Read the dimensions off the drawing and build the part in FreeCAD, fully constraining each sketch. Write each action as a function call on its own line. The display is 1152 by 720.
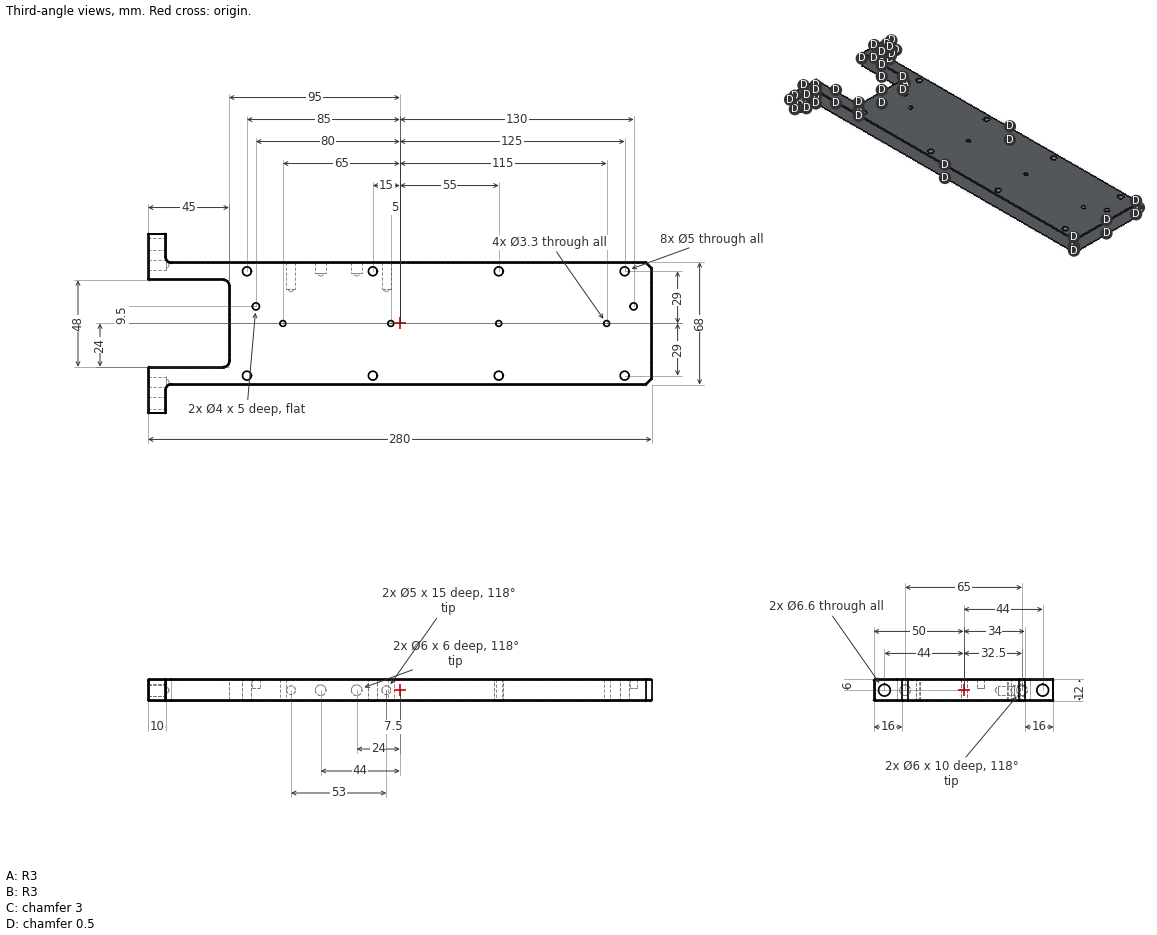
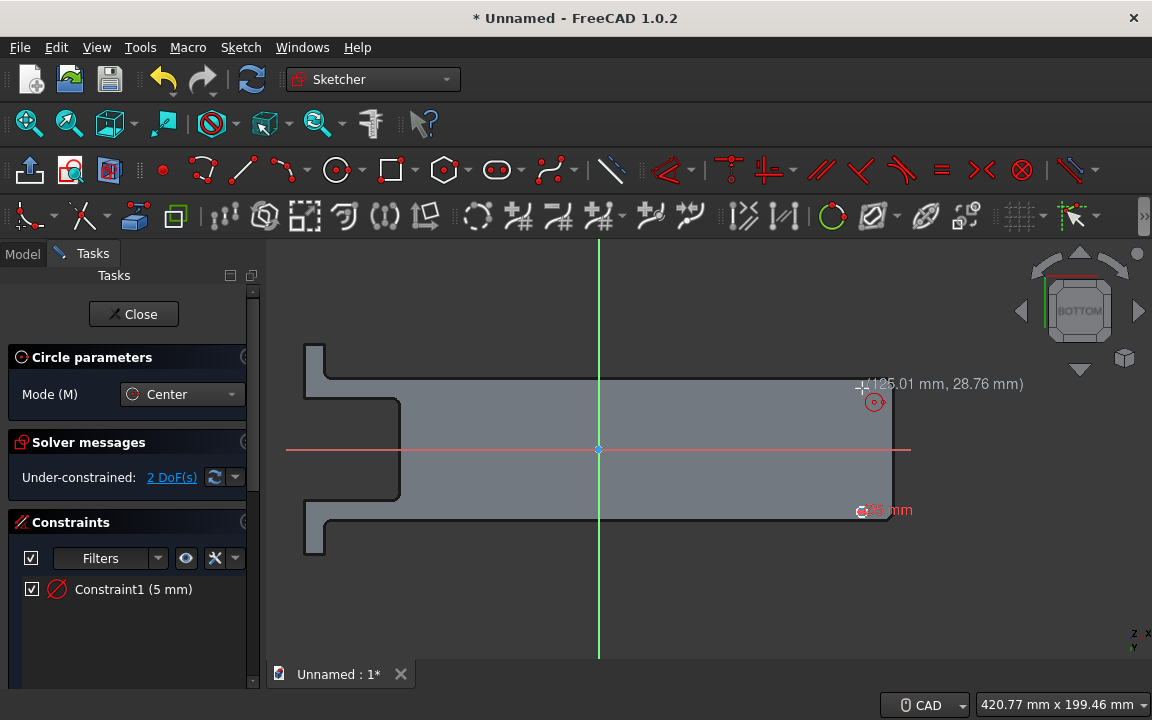
click(862, 388)
move(866, 385)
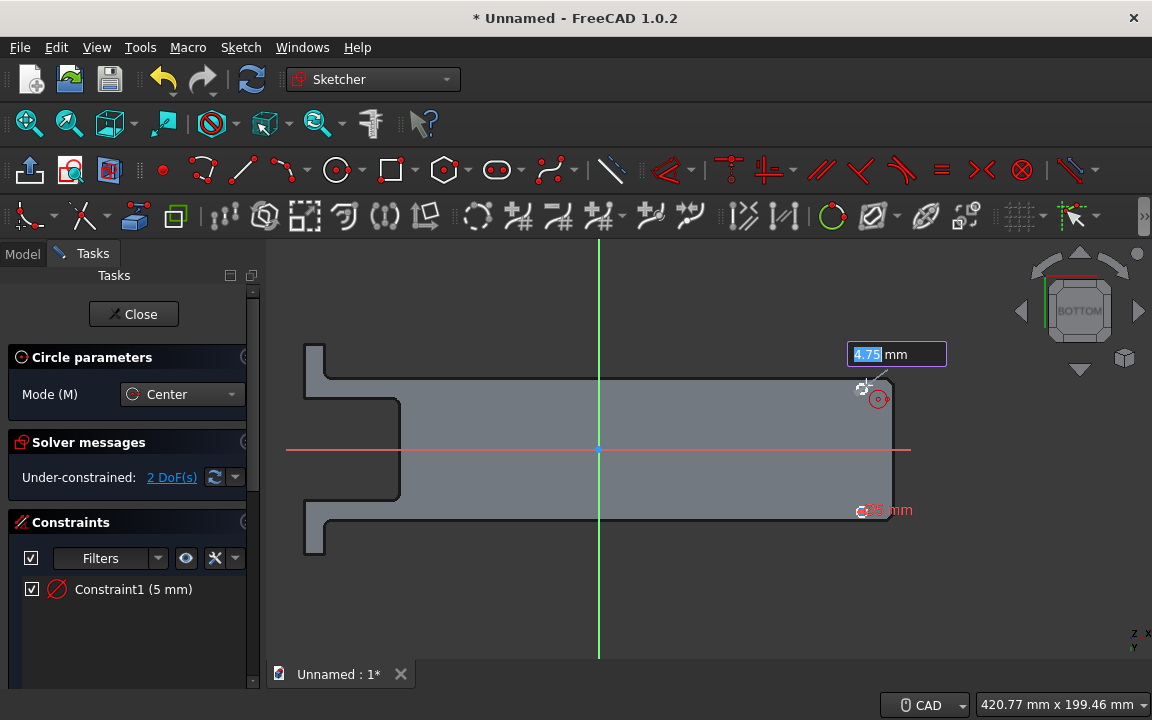
text(5)
key(Return)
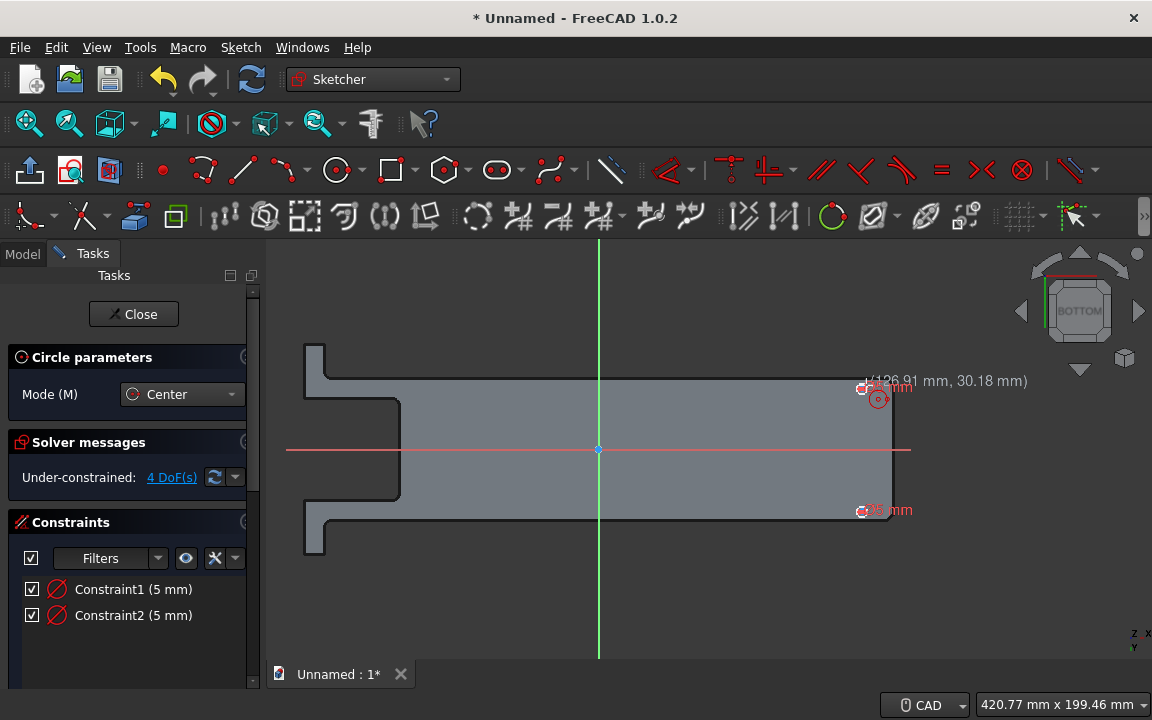
scroll(715, 511, up, 8)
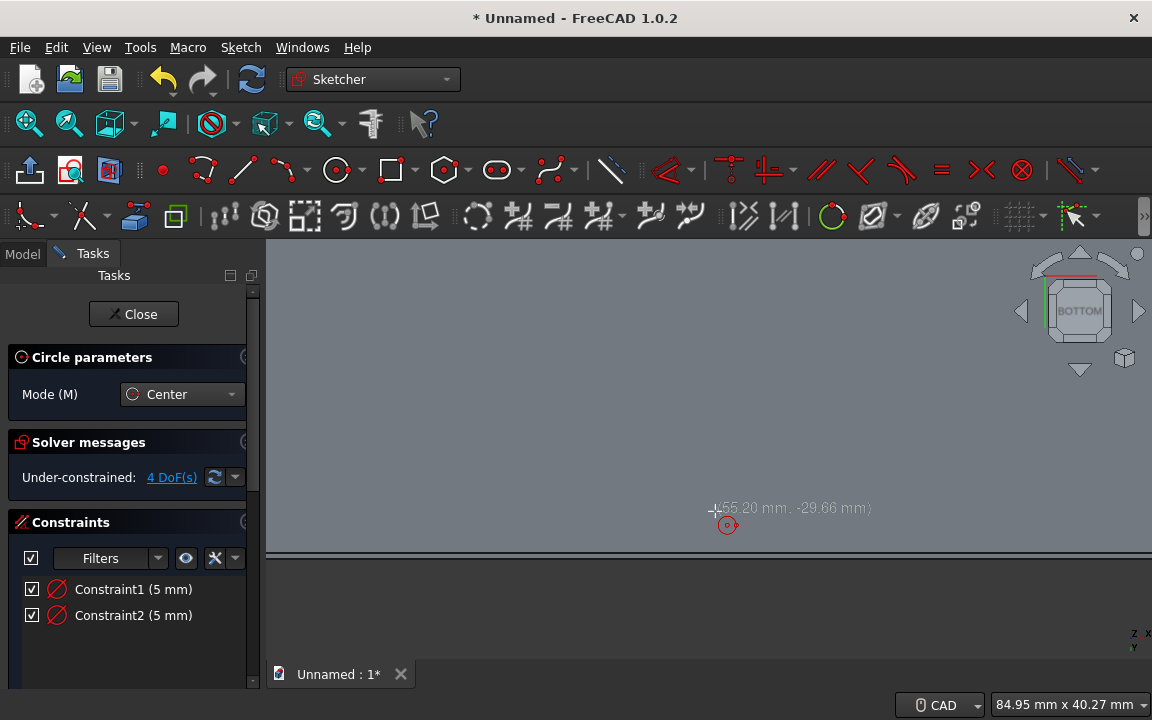
scroll(715, 511, down, 8)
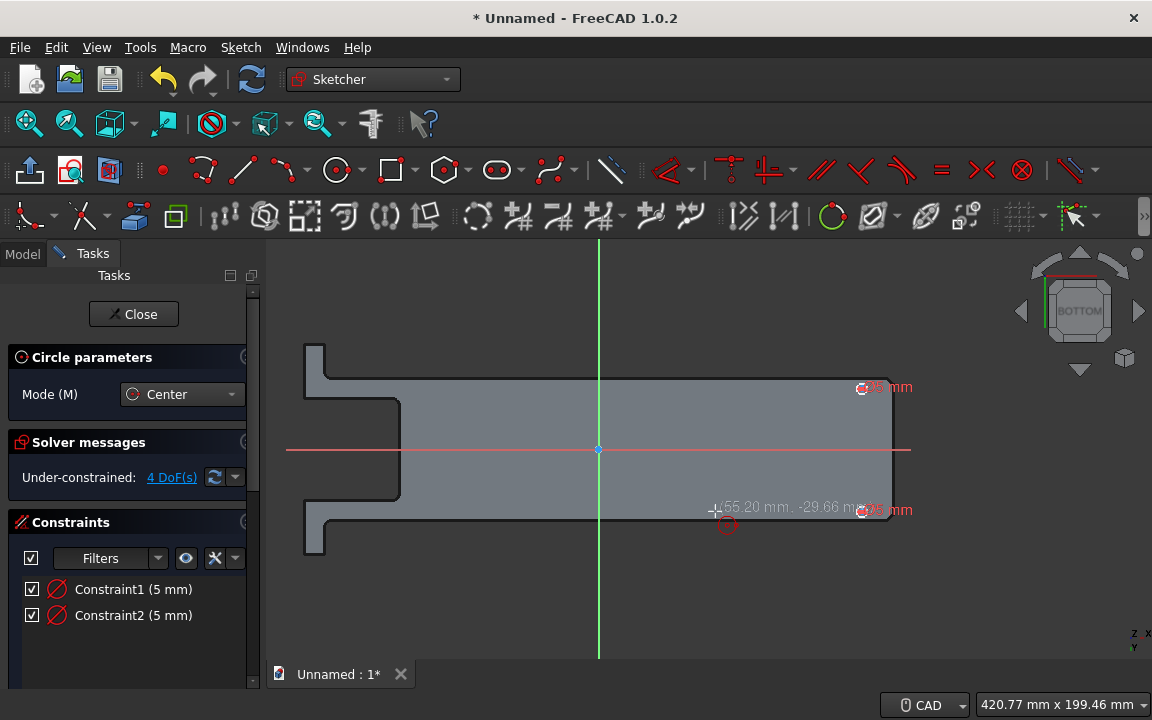
click(715, 511)
move(718, 507)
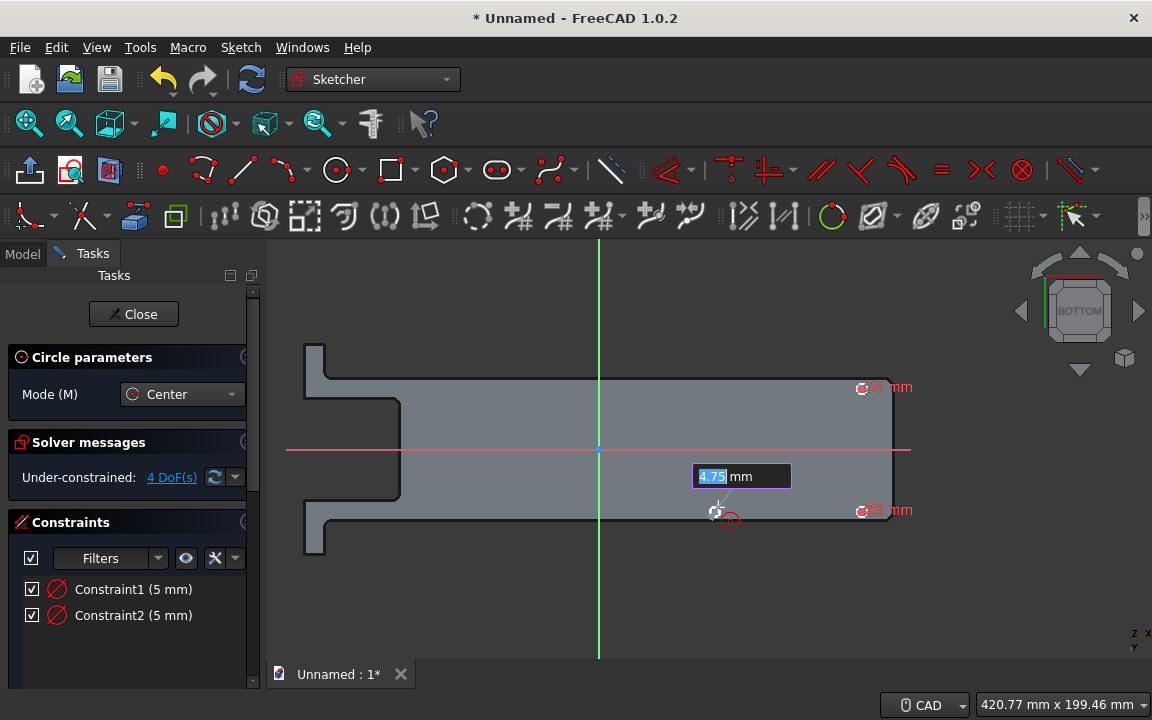
text(5)
key(Return)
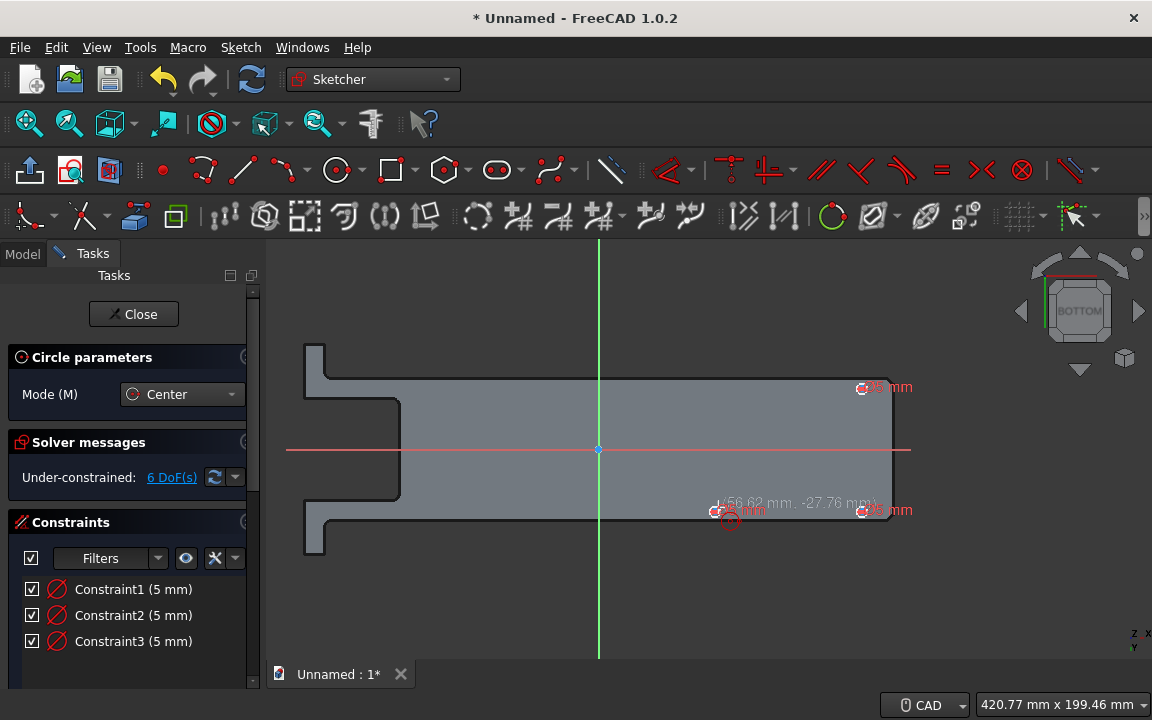
scroll(715, 388, up, 8)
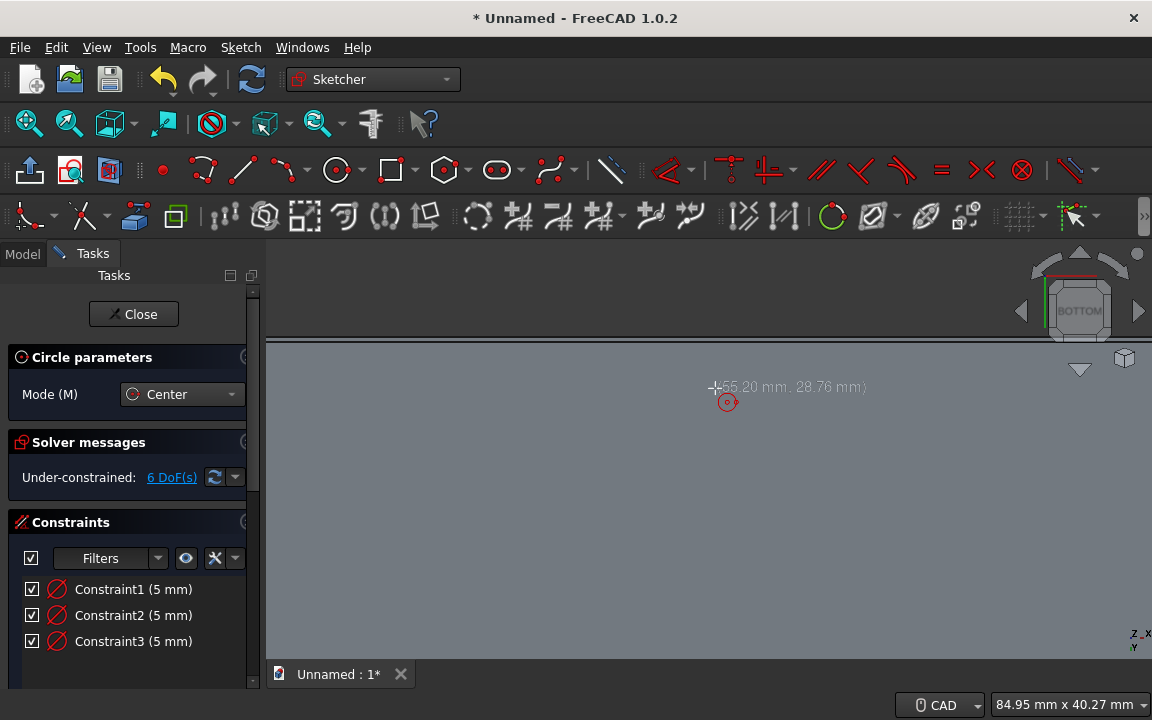
scroll(715, 388, down, 8)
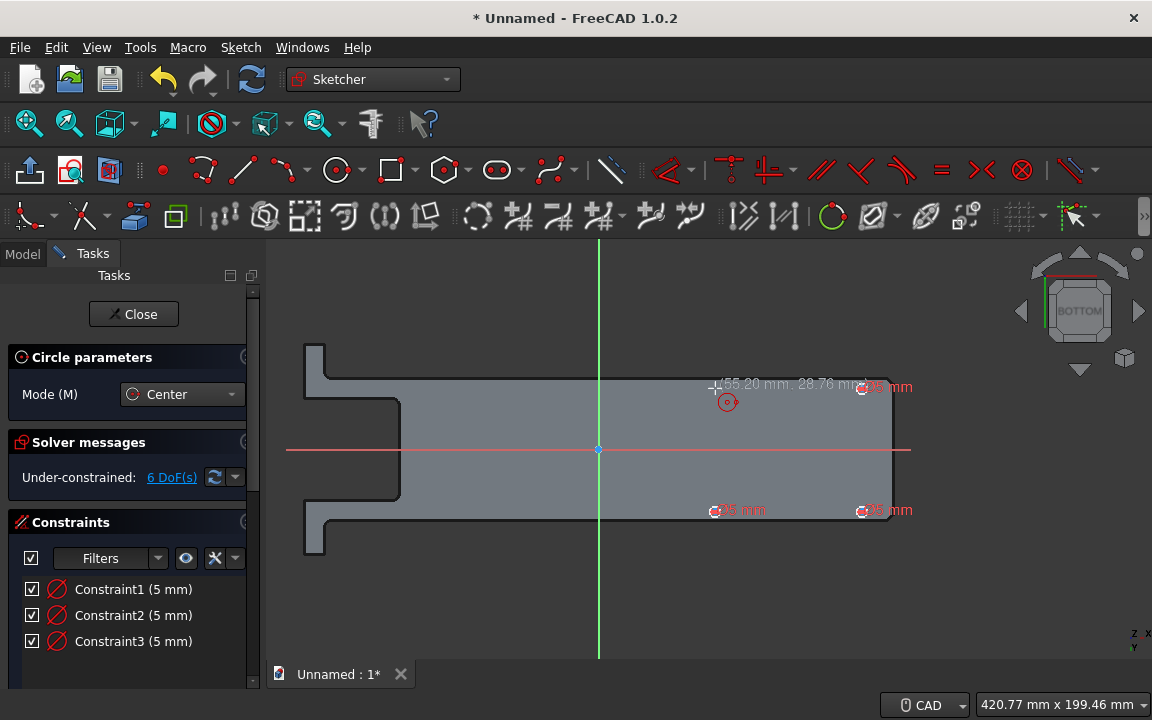
click(715, 388)
move(718, 385)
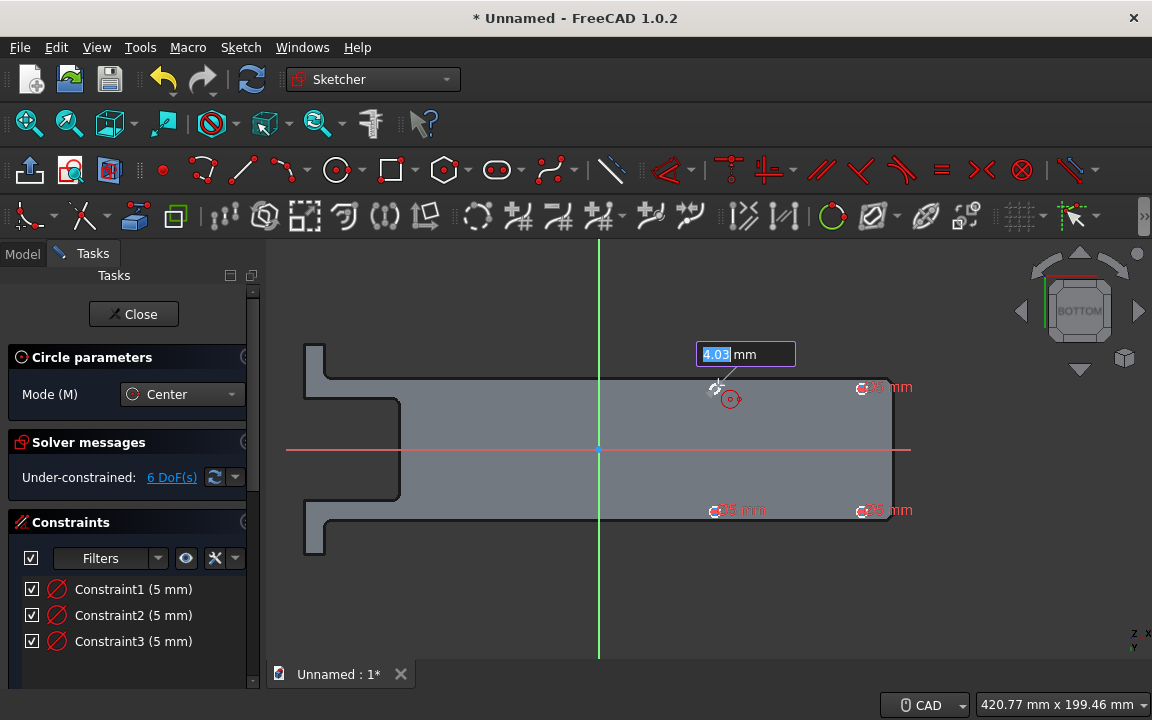
text(5)
key(Return)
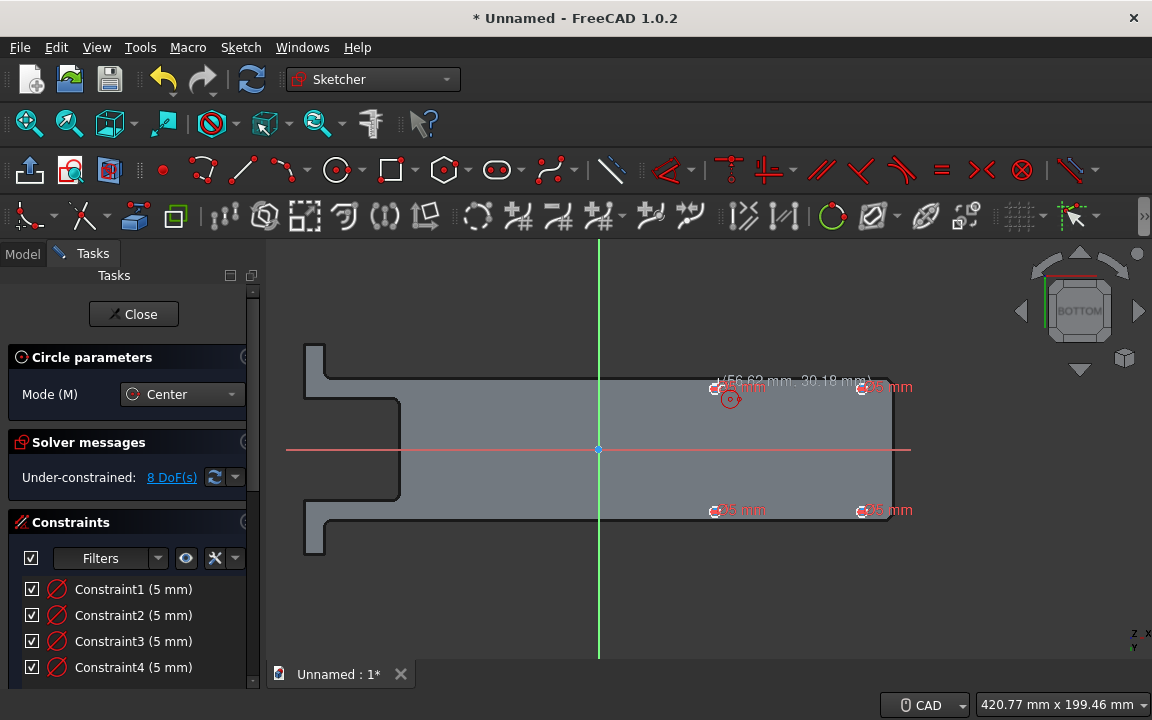
scroll(567, 511, up, 8)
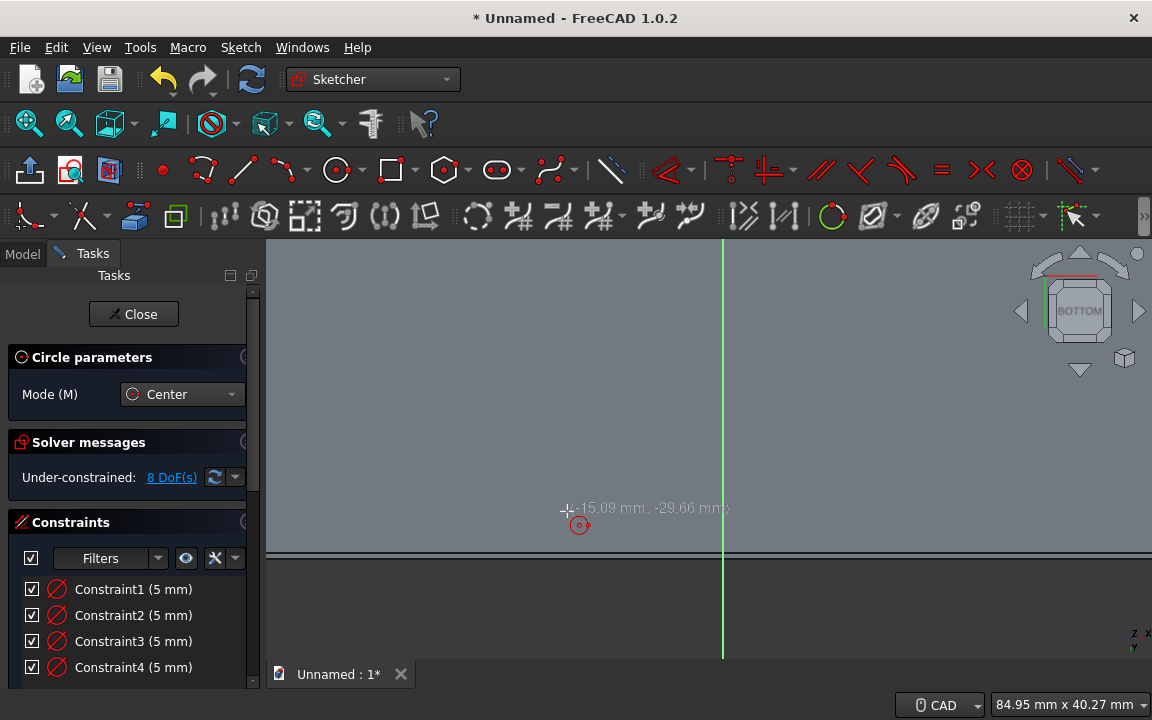
scroll(567, 511, down, 8)